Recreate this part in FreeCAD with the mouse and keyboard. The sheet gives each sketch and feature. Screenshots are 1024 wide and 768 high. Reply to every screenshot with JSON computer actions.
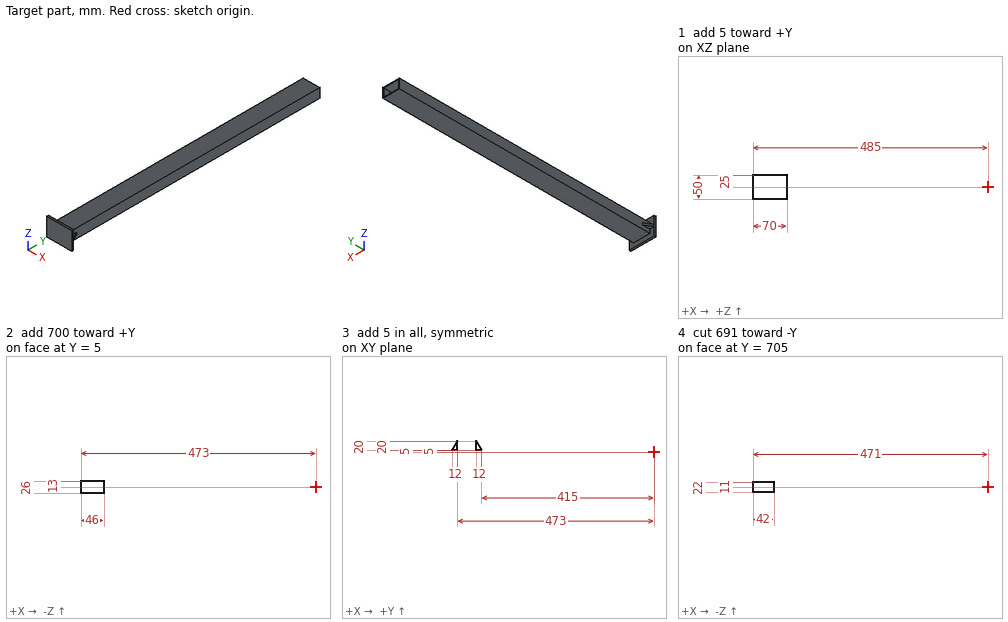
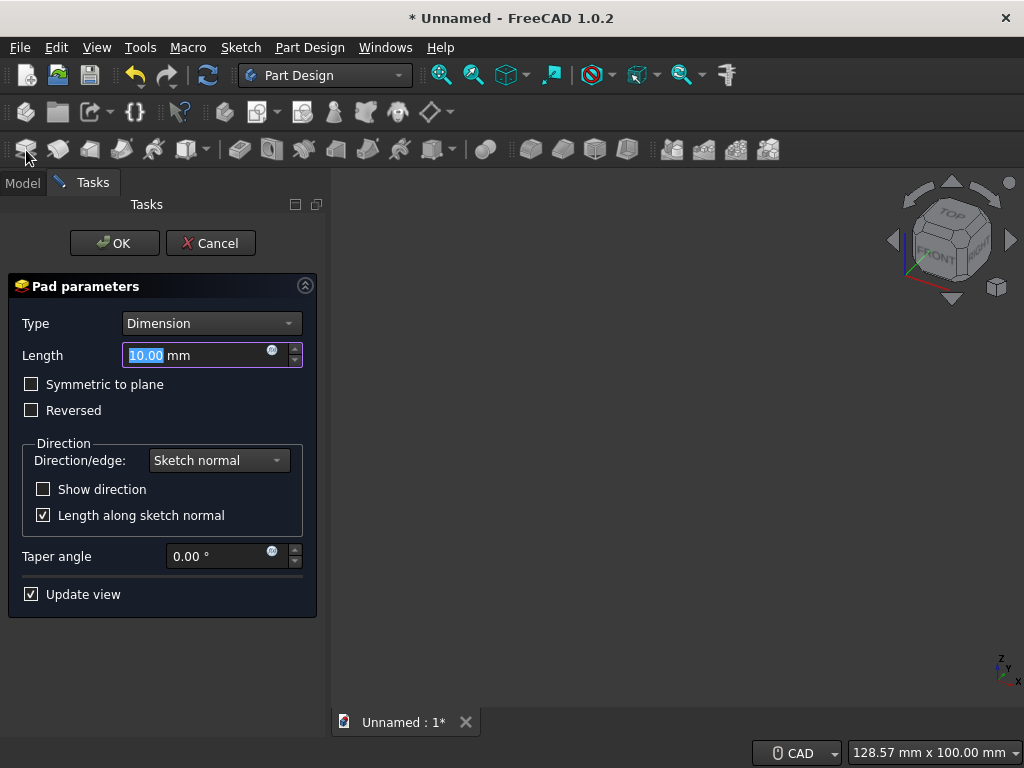
{"action": "type", "text": "5"}
{"action": "key", "text": "Tab"}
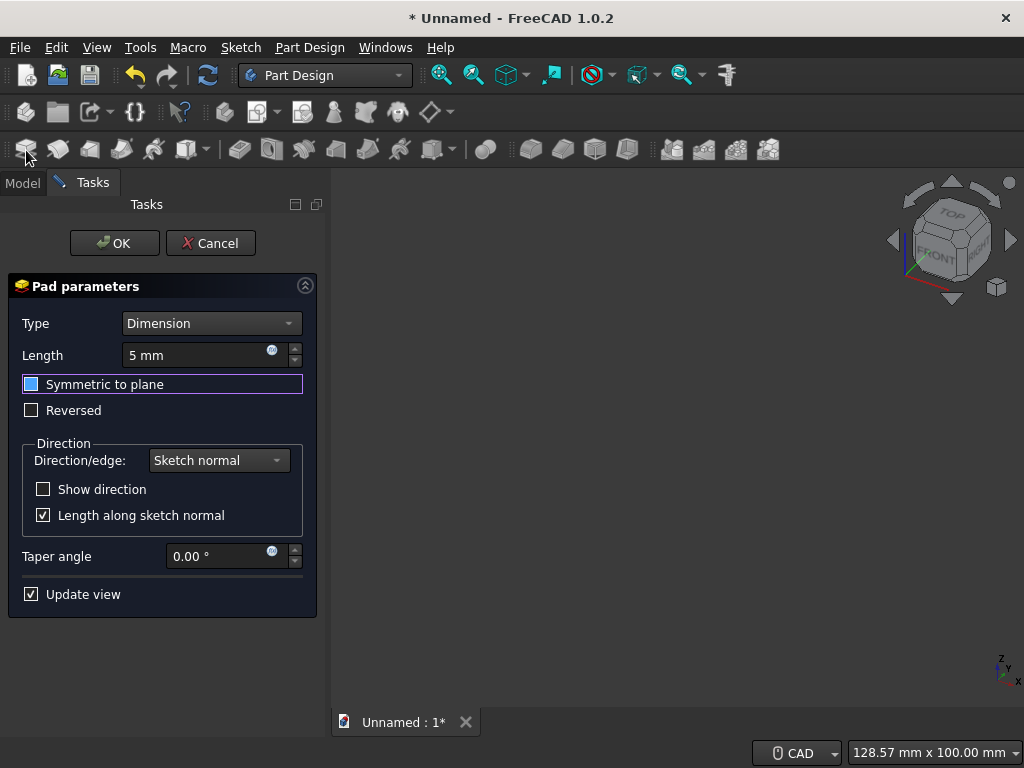
{"action": "left_click", "coordinate": [30, 410]}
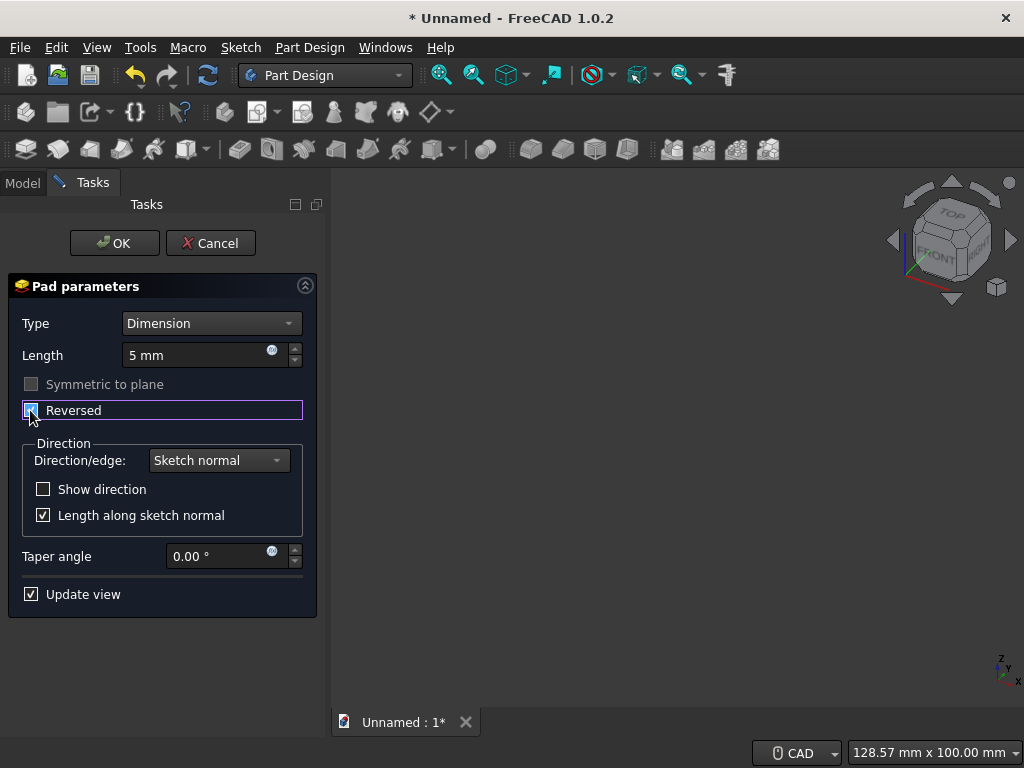
{"action": "left_click", "coordinate": [115, 243]}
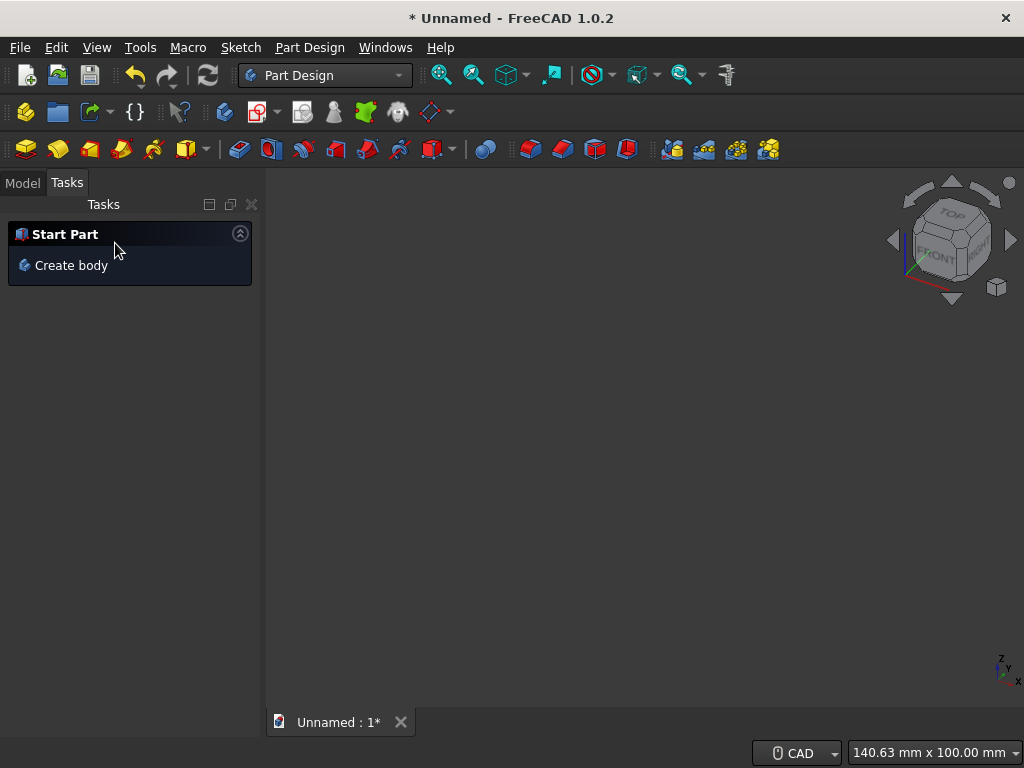
{"action": "left_click", "coordinate": [442, 76]}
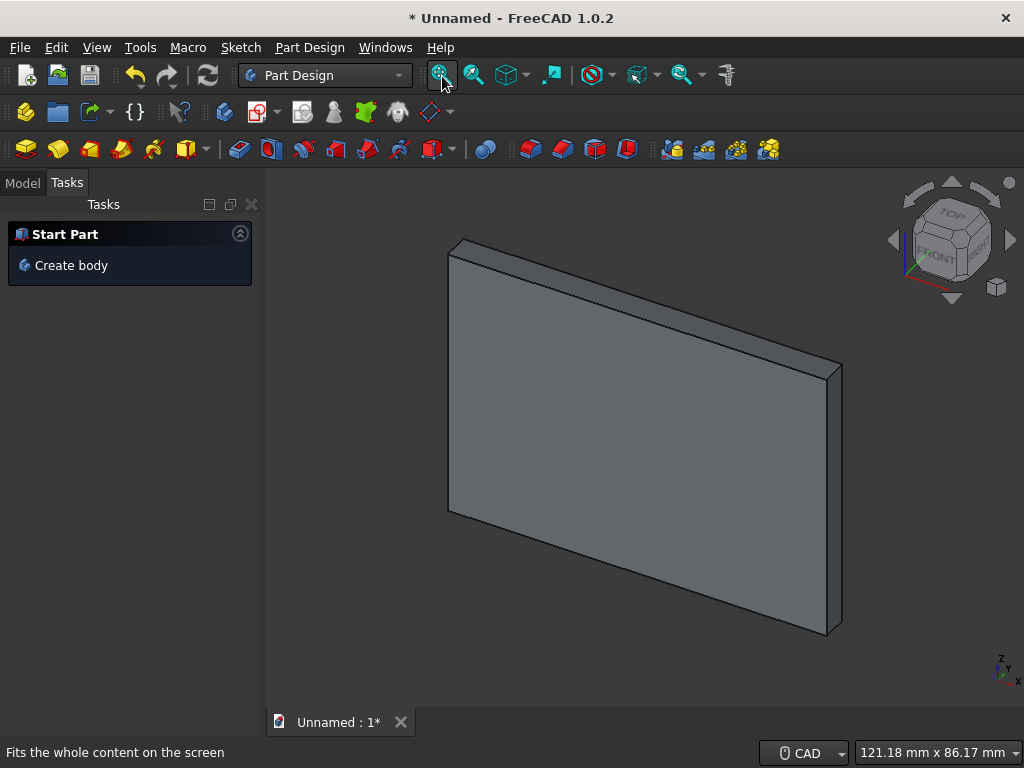
{"action": "key", "text": "4"}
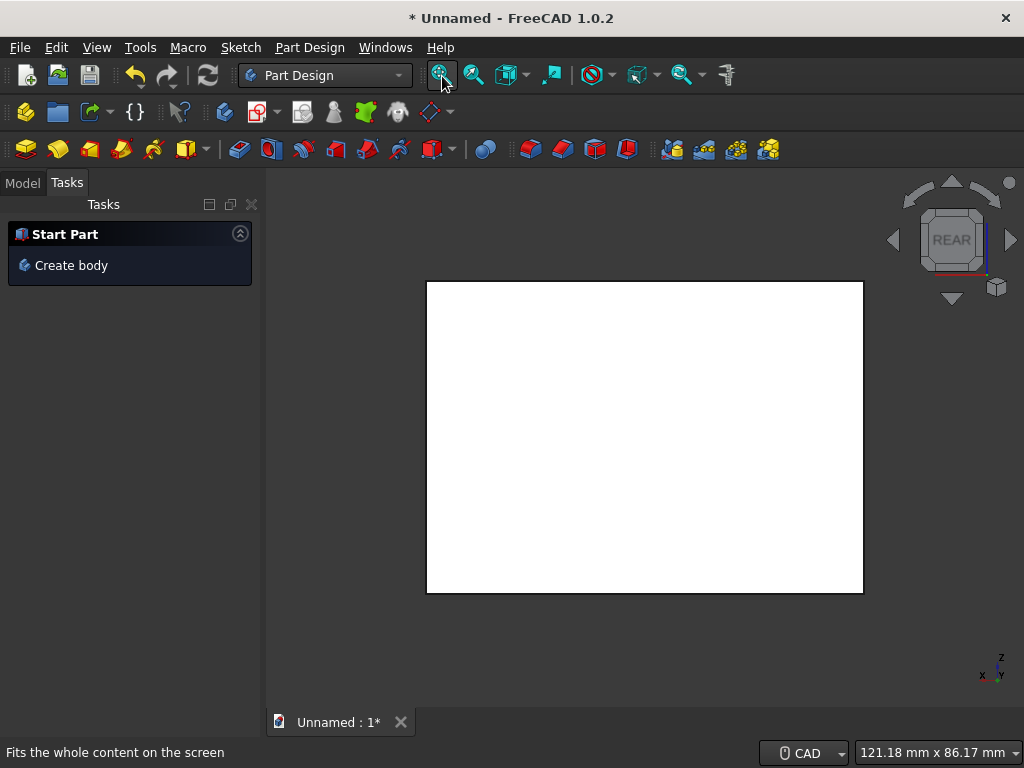
{"action": "left_click", "coordinate": [645, 436]}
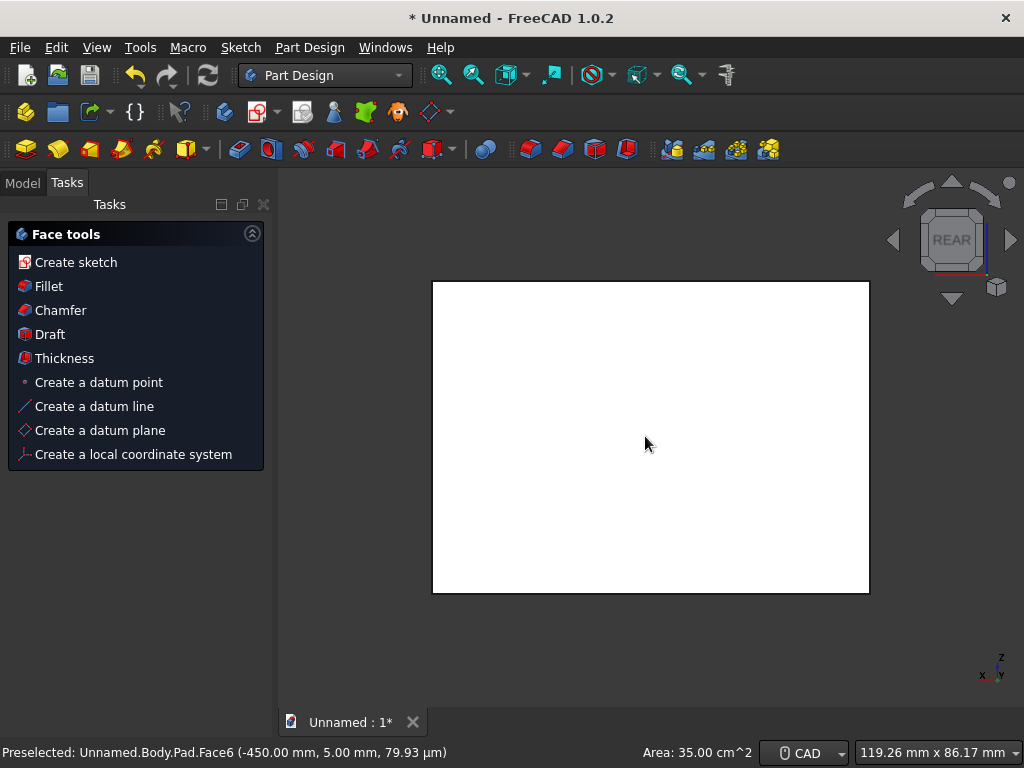
{"action": "left_click", "coordinate": [258, 112]}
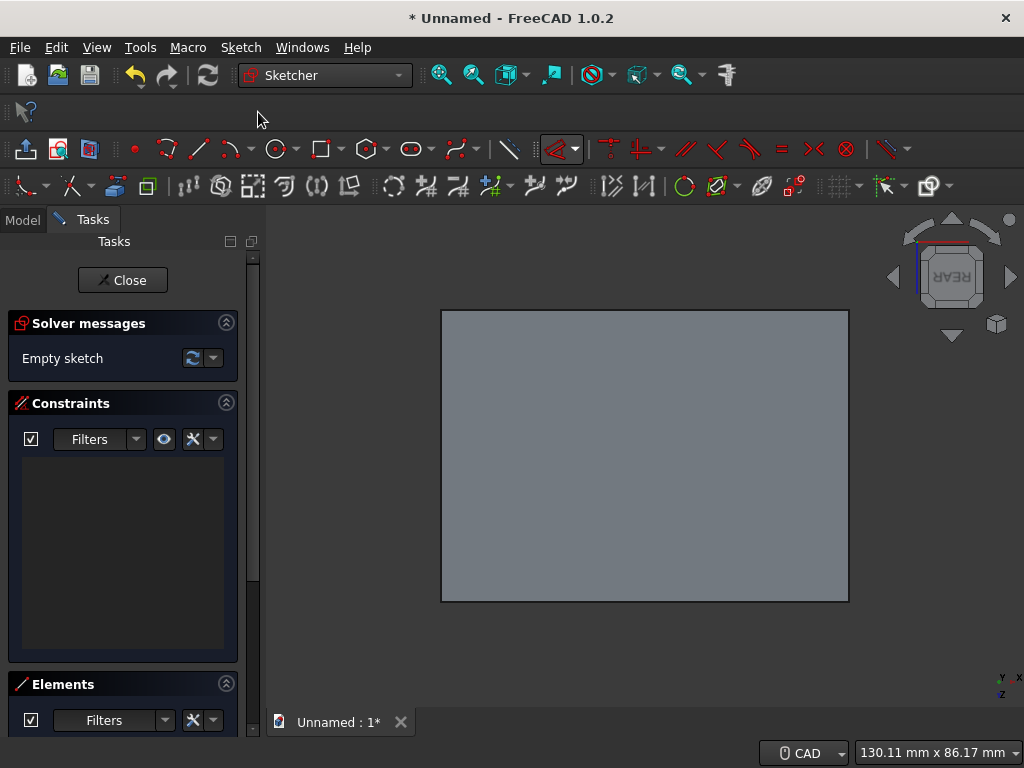
{"action": "scroll", "coordinate": [784, 456], "scroll_direction": "up", "scroll_amount": 2}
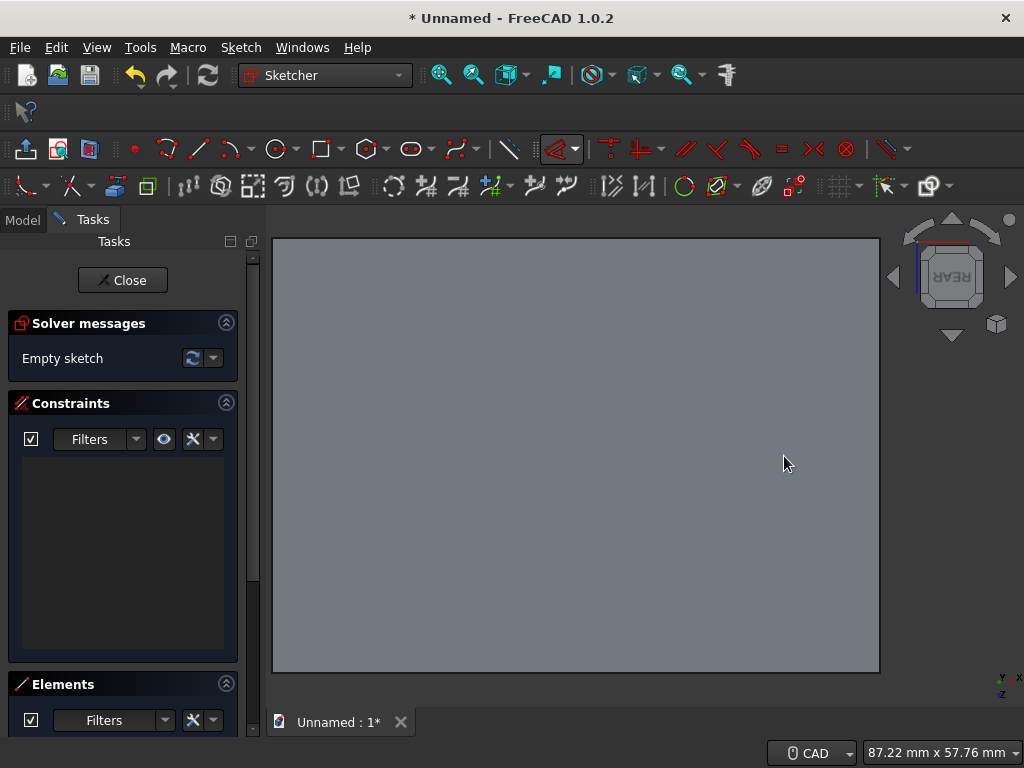
{"action": "key", "text": "g r"}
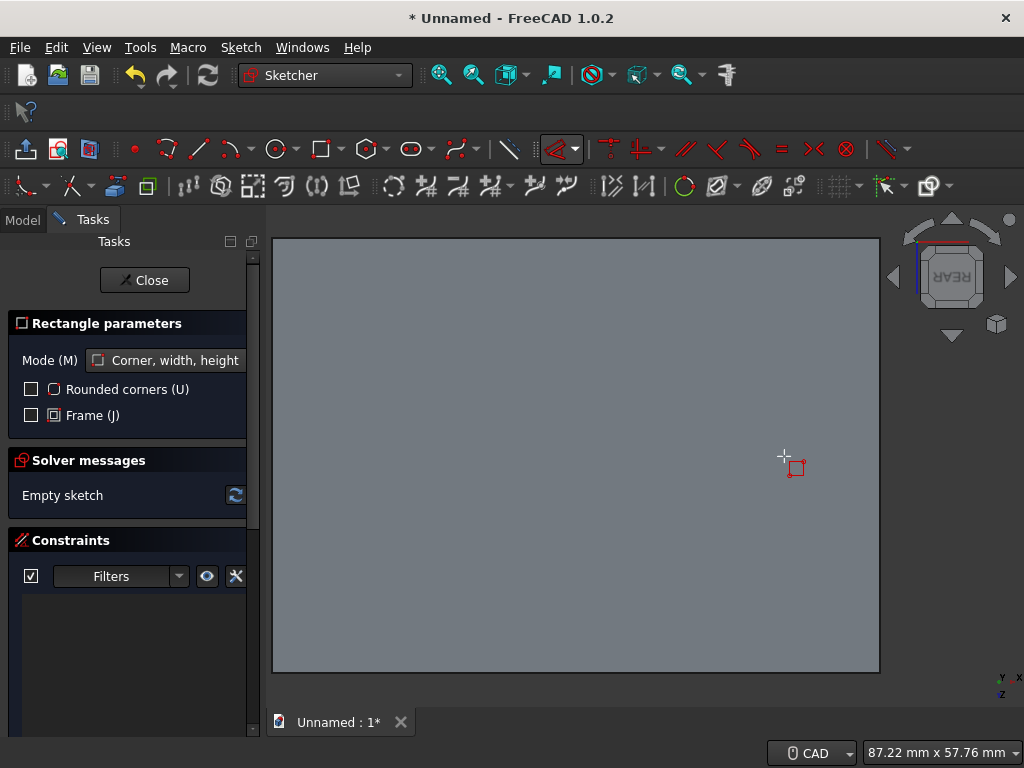
{"action": "left_click", "coordinate": [376, 343]}
{"action": "left_click", "coordinate": [776, 569]}
{"action": "key", "text": "Escape"}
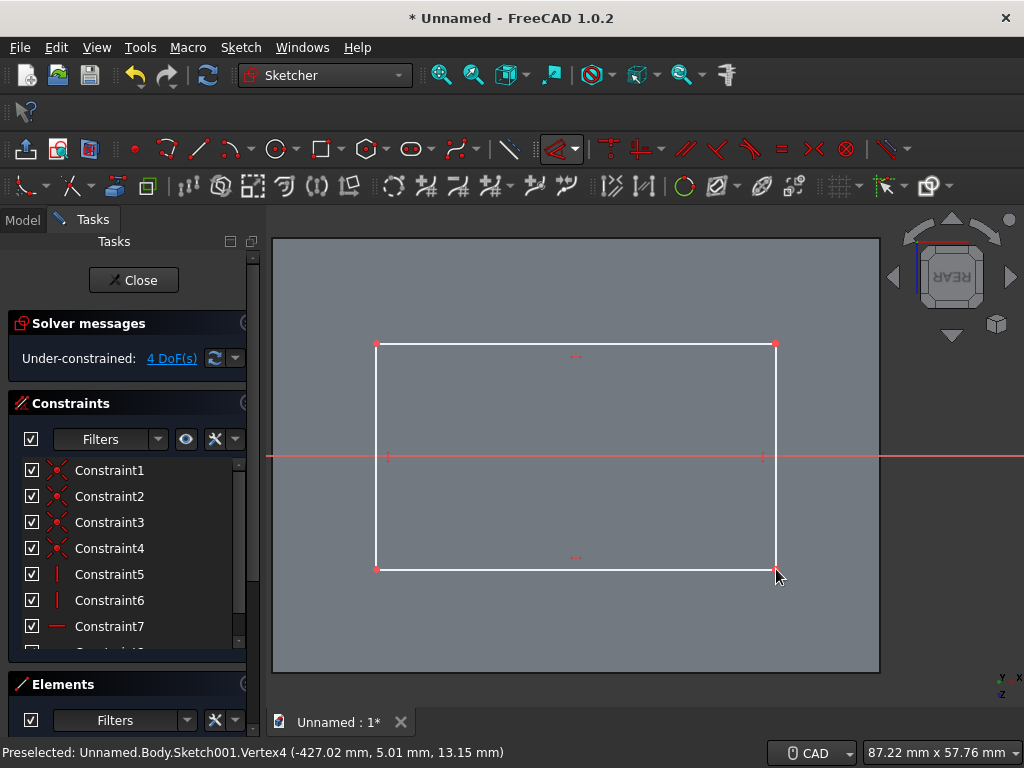
{"action": "left_click", "coordinate": [376, 412]}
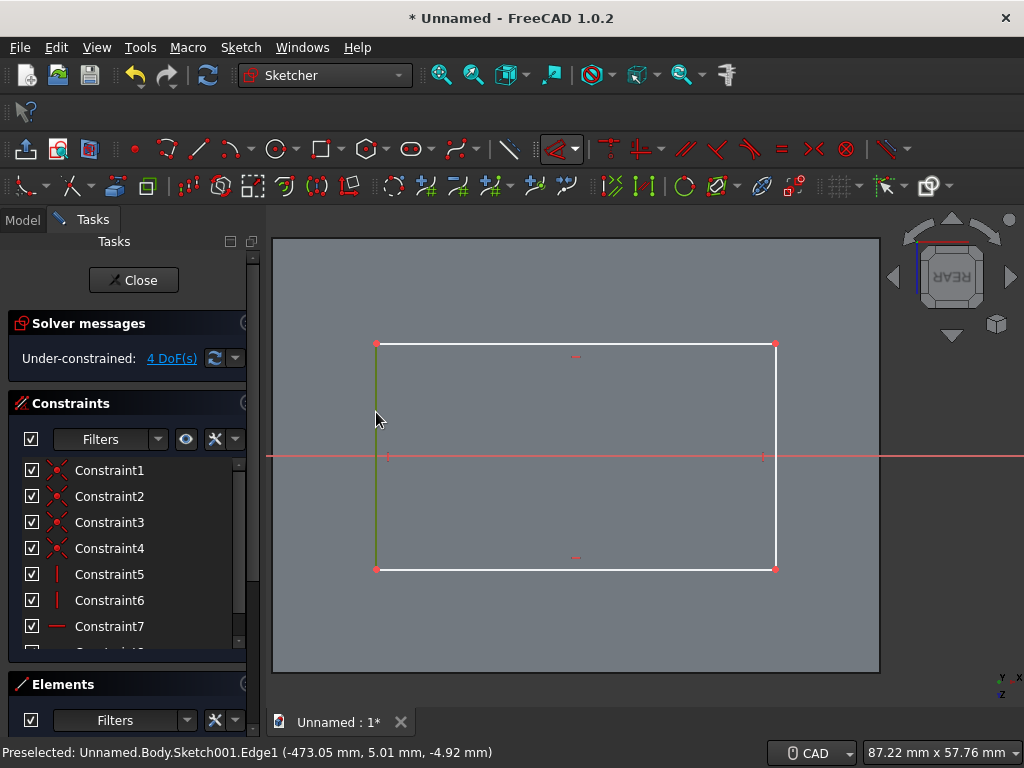
{"action": "key", "text": "i"}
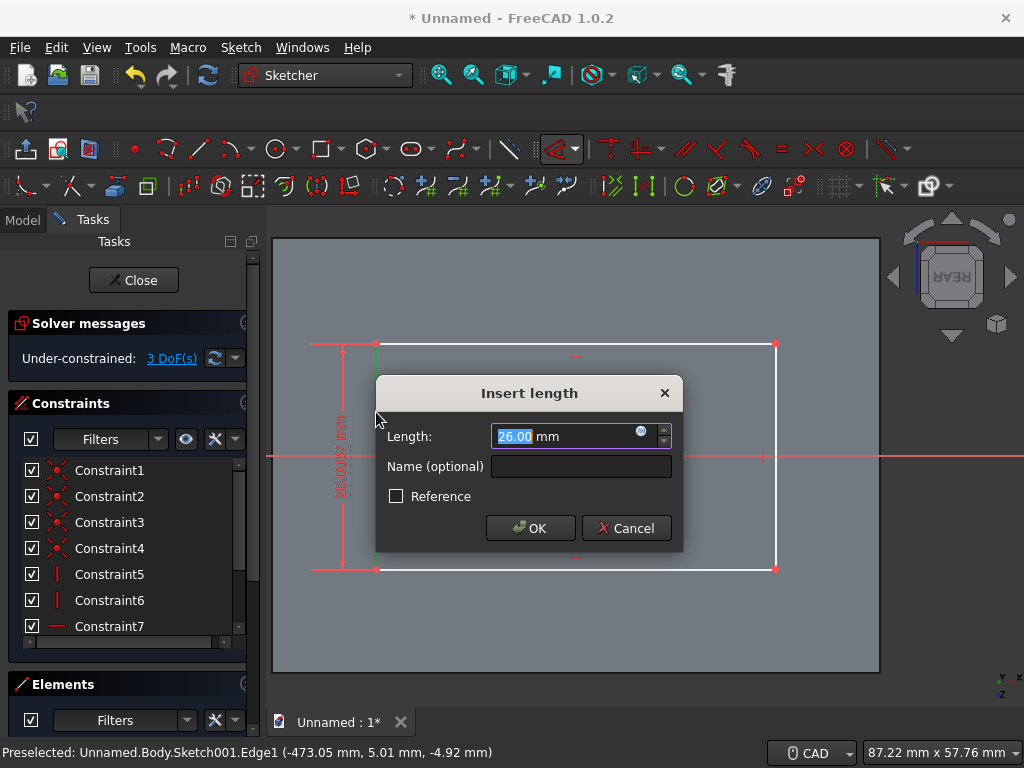
{"action": "type", "text": "26"}
{"action": "key", "text": "Return"}